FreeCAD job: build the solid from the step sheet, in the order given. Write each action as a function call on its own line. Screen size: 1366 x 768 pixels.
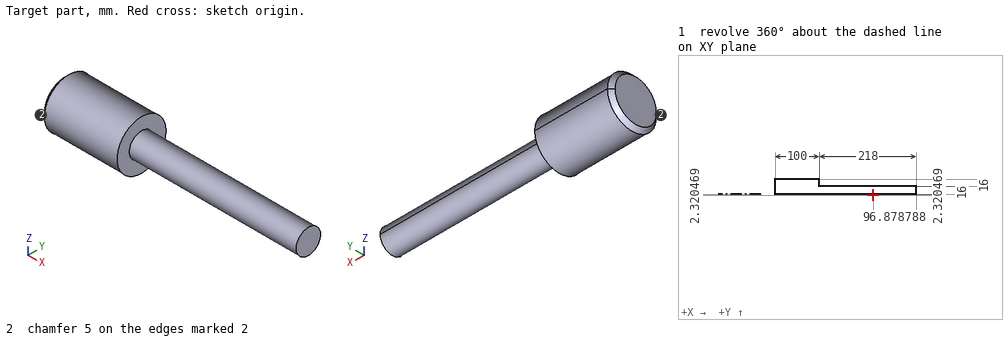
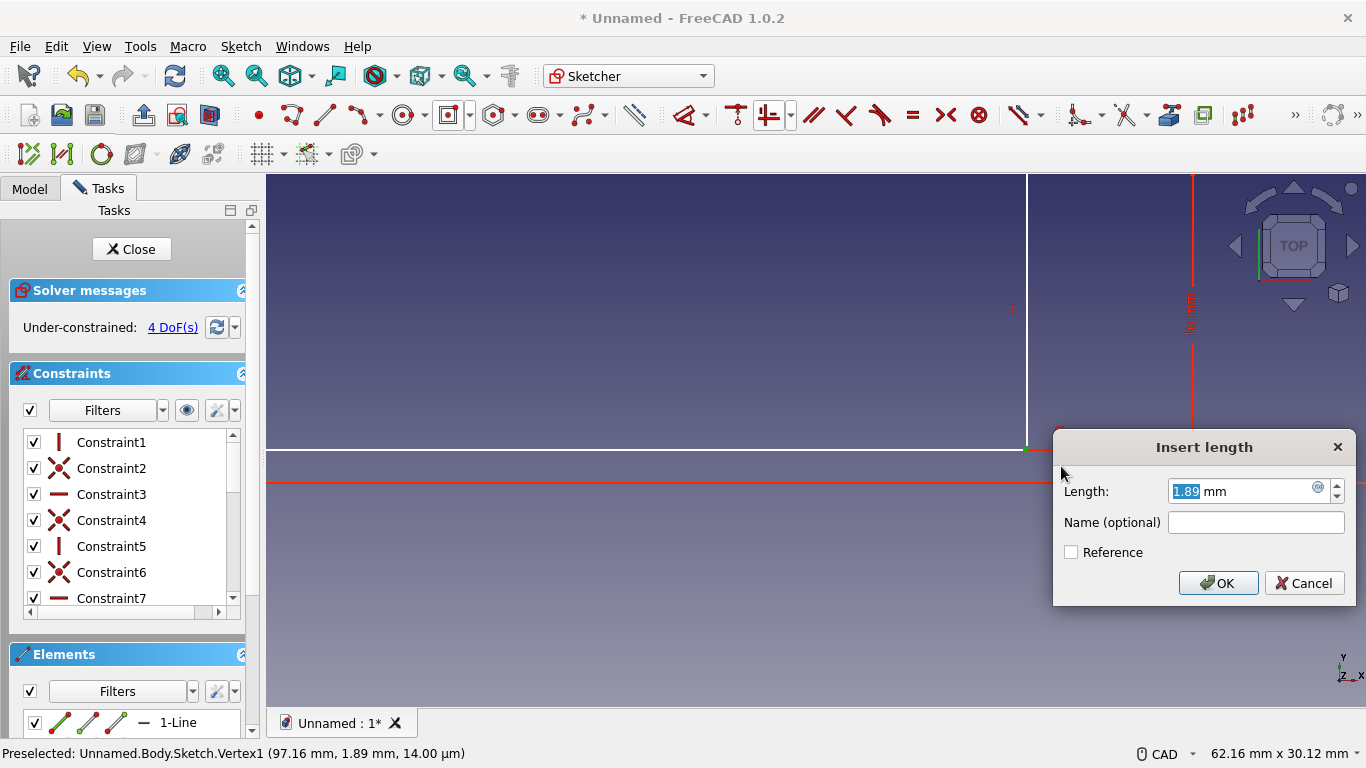
text(2.320469)
key(Return)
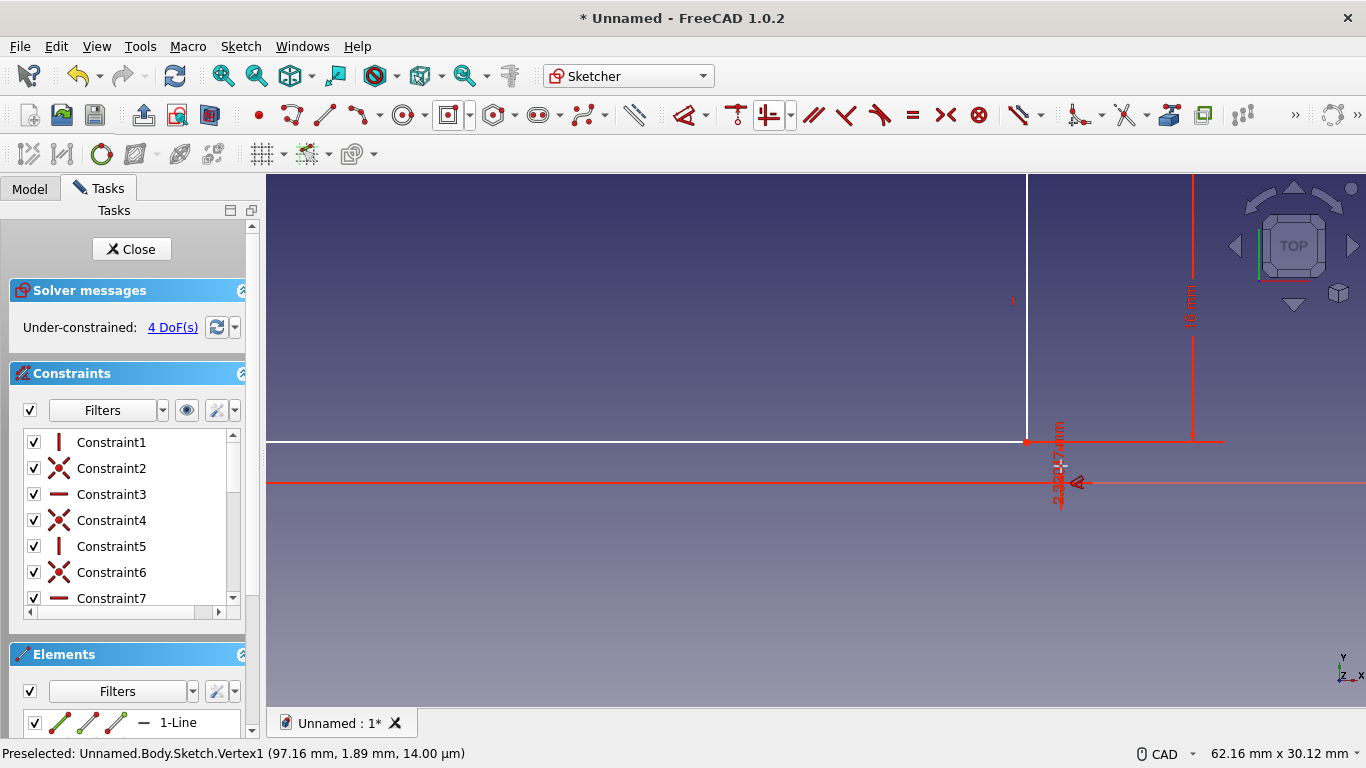
scroll(1042, 461, down, 13)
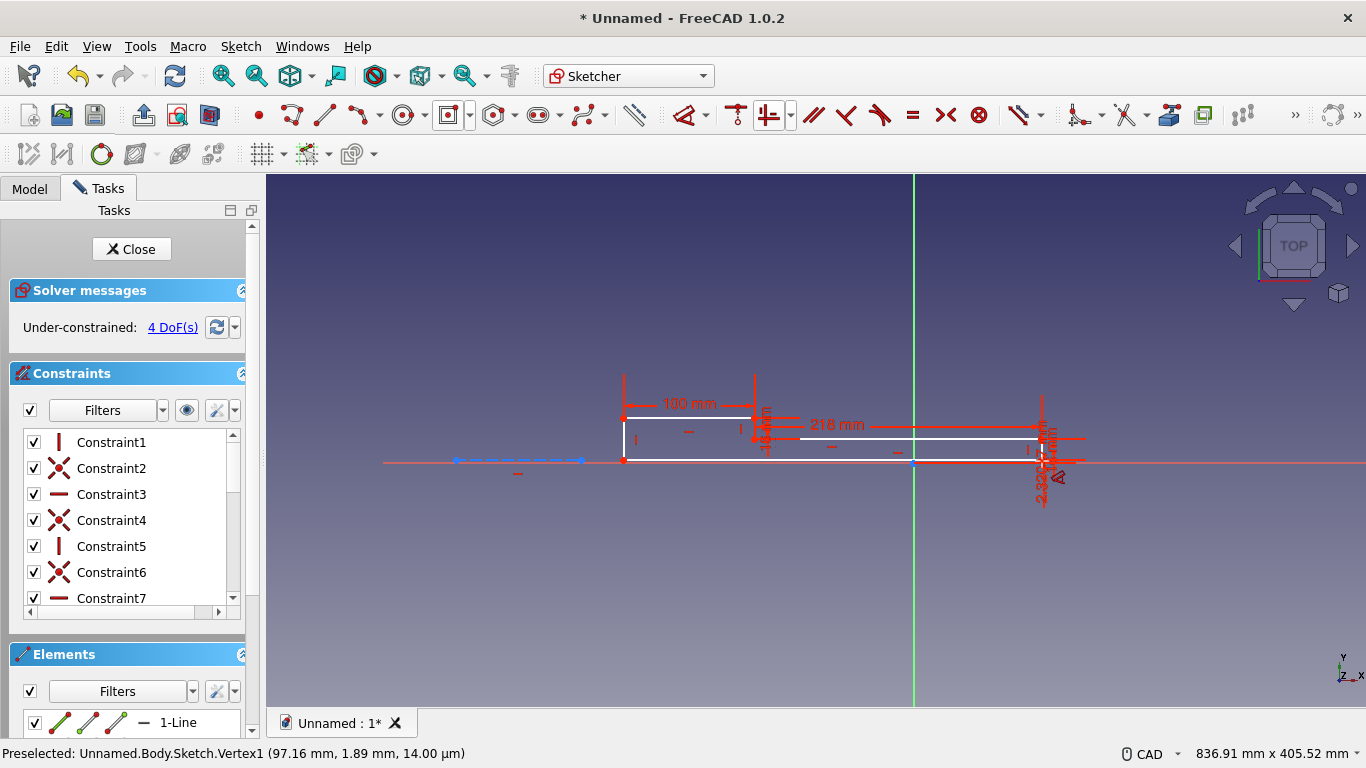
scroll(581, 460, up, 13)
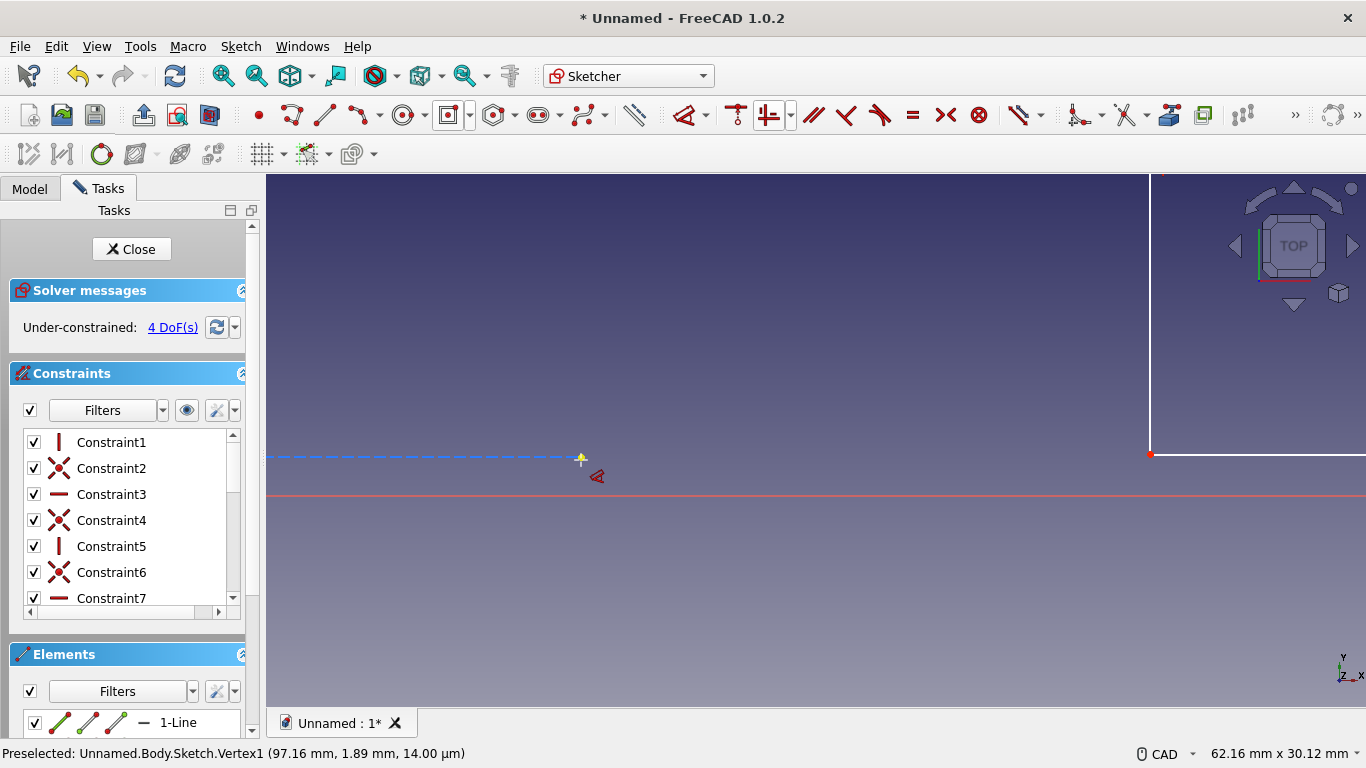
click(582, 457)
click(548, 476)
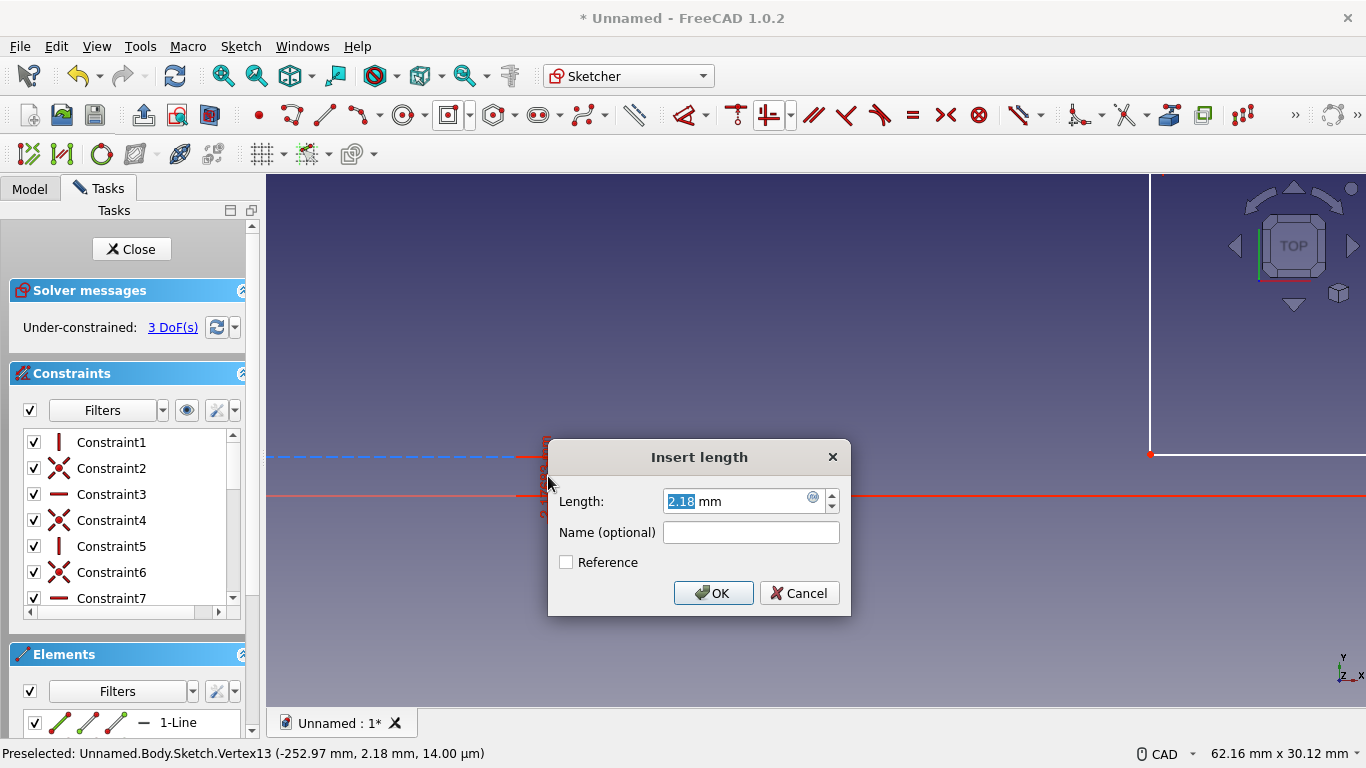
text(2.320469)
key(Return)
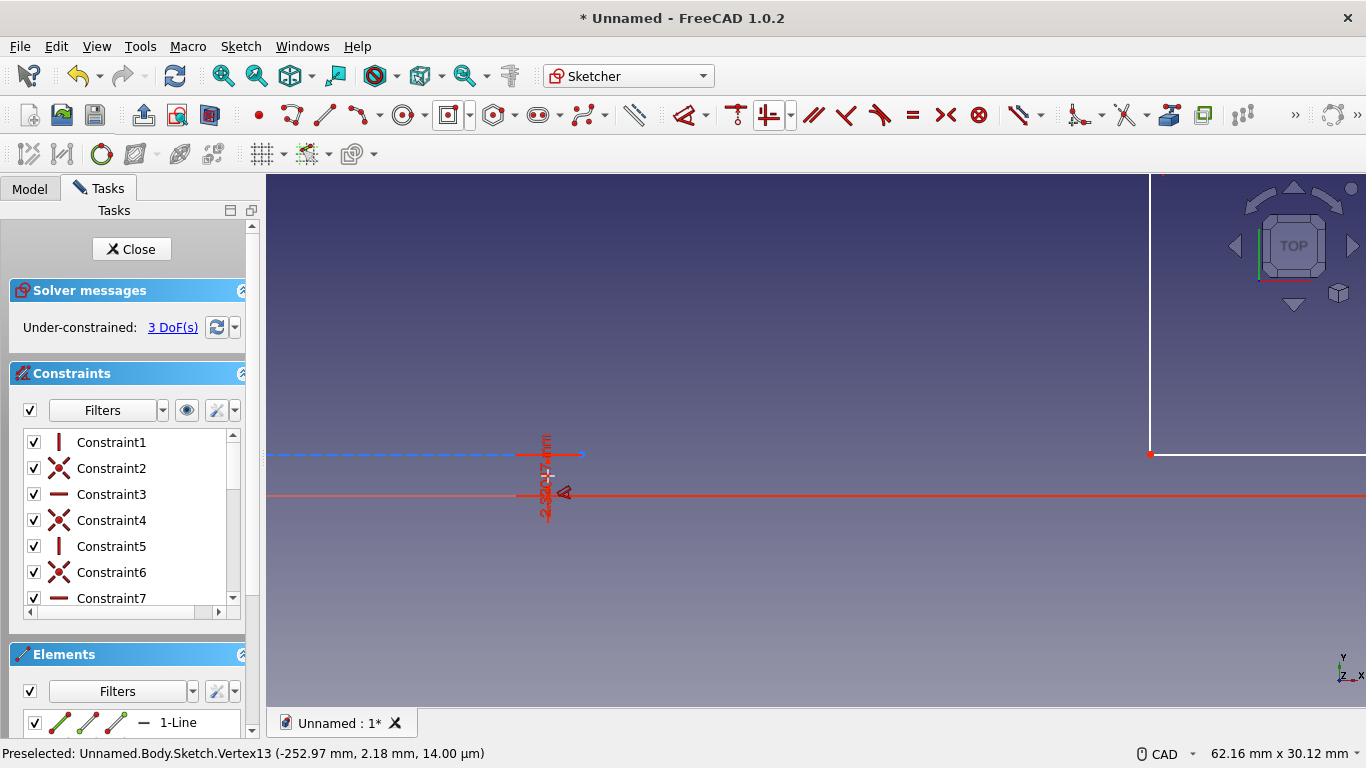
scroll(580, 460, down, 13)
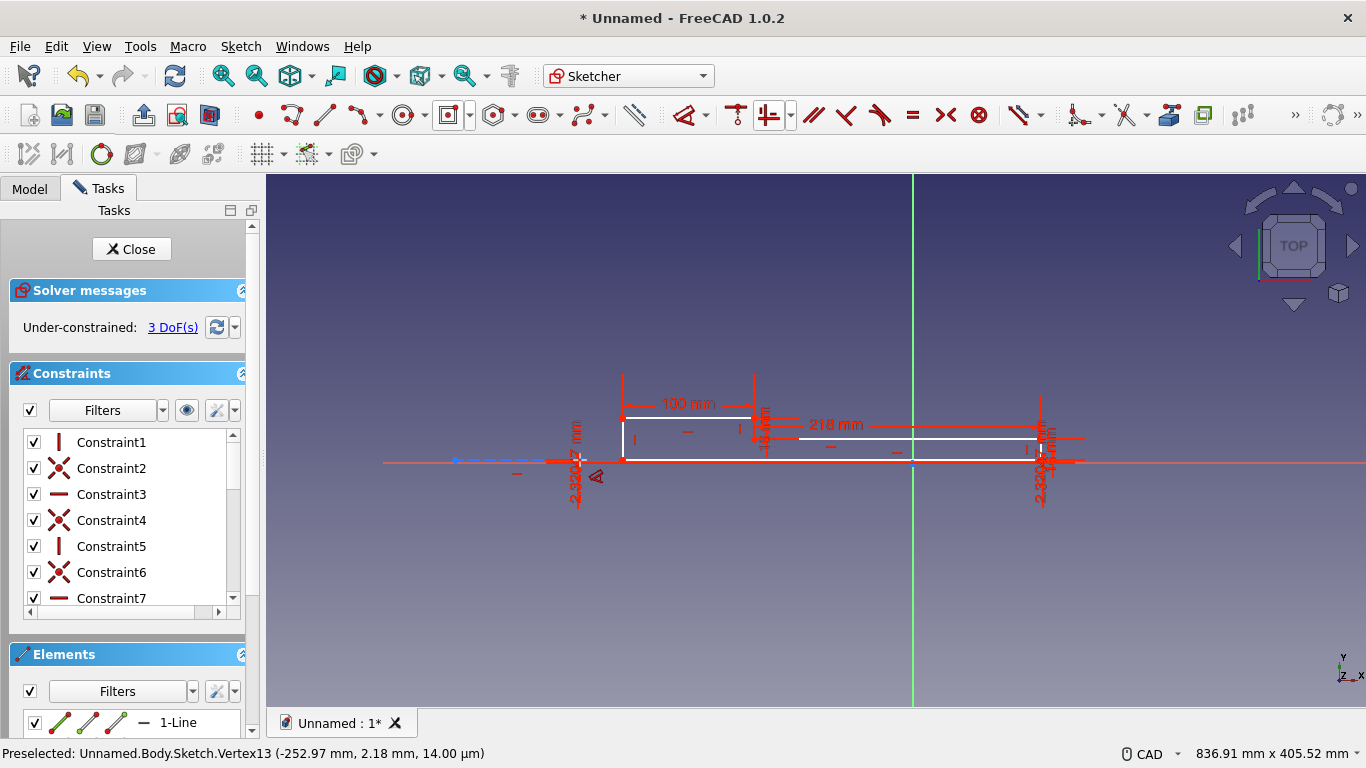
click(1041, 460)
click(977, 497)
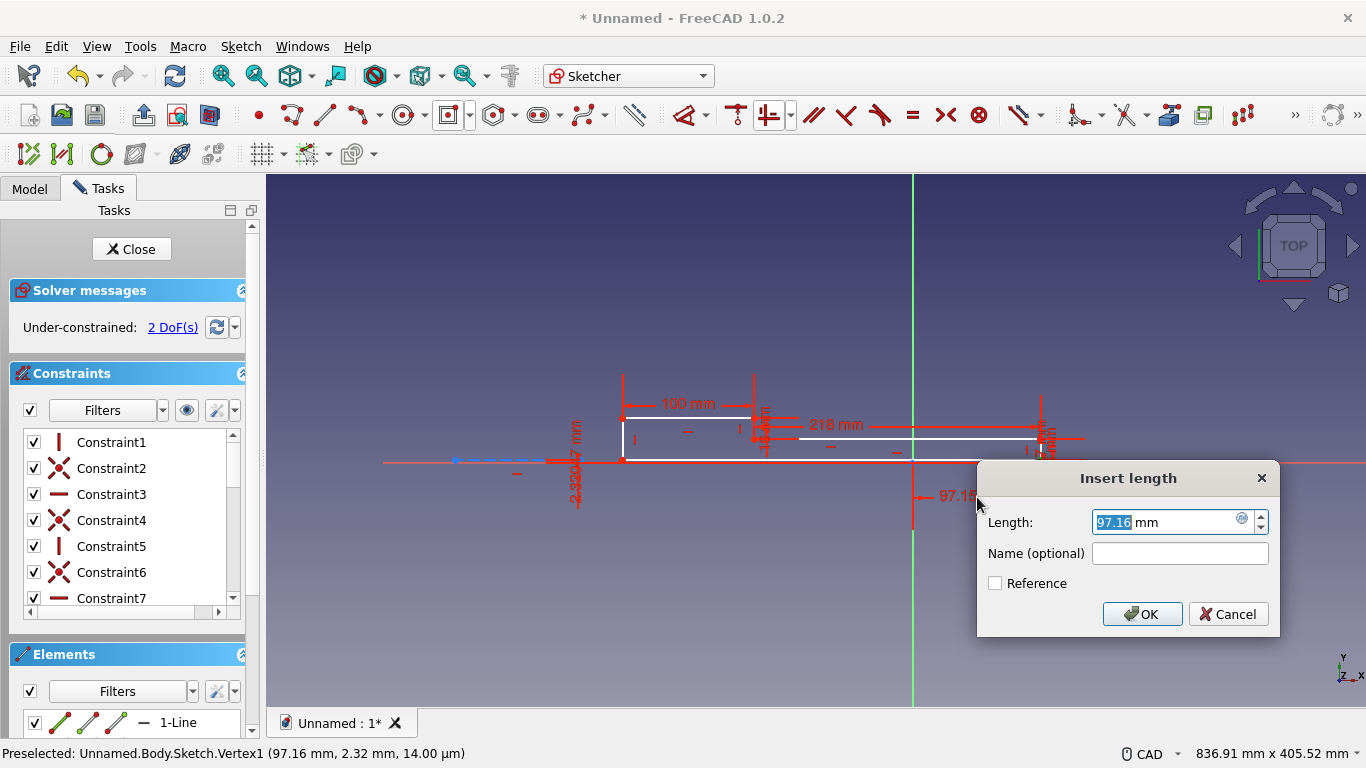
text(96.878788)
key(Return)
key(Escape)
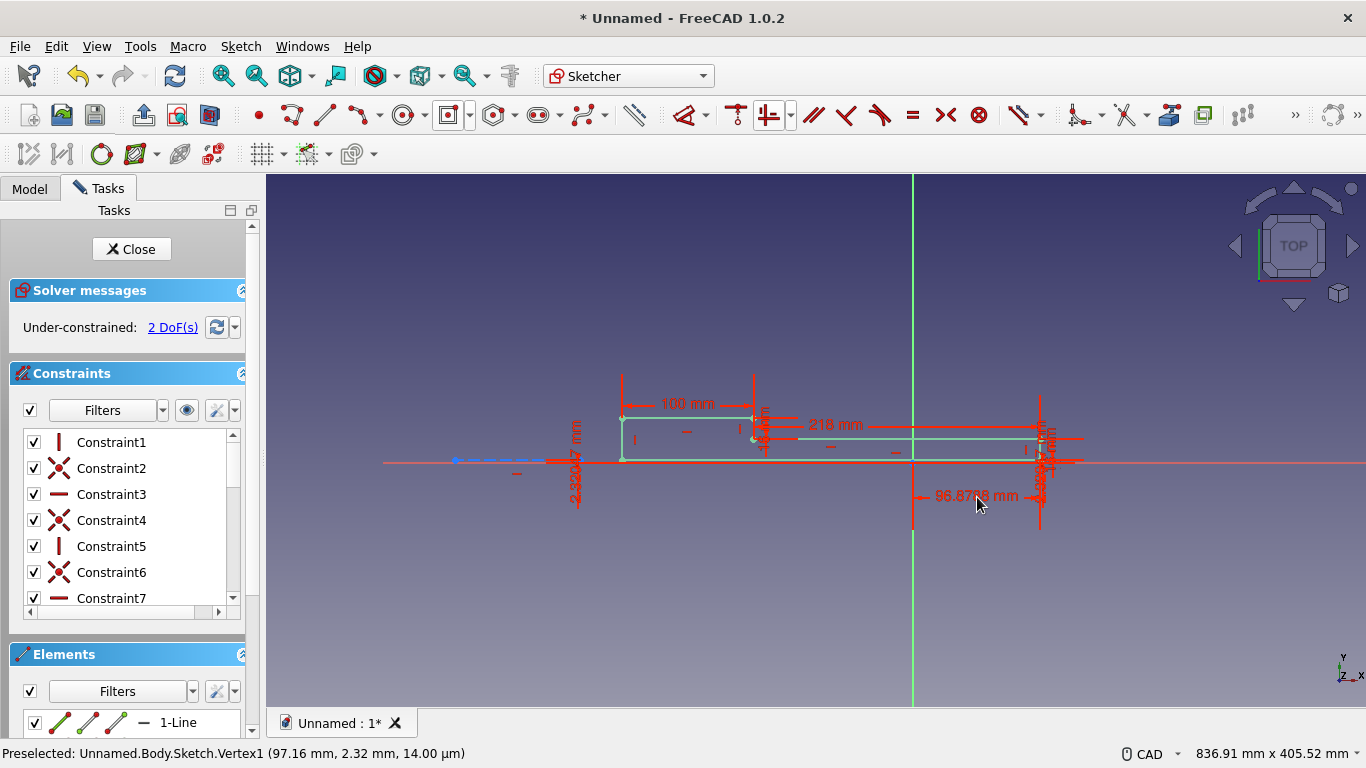
click(132, 249)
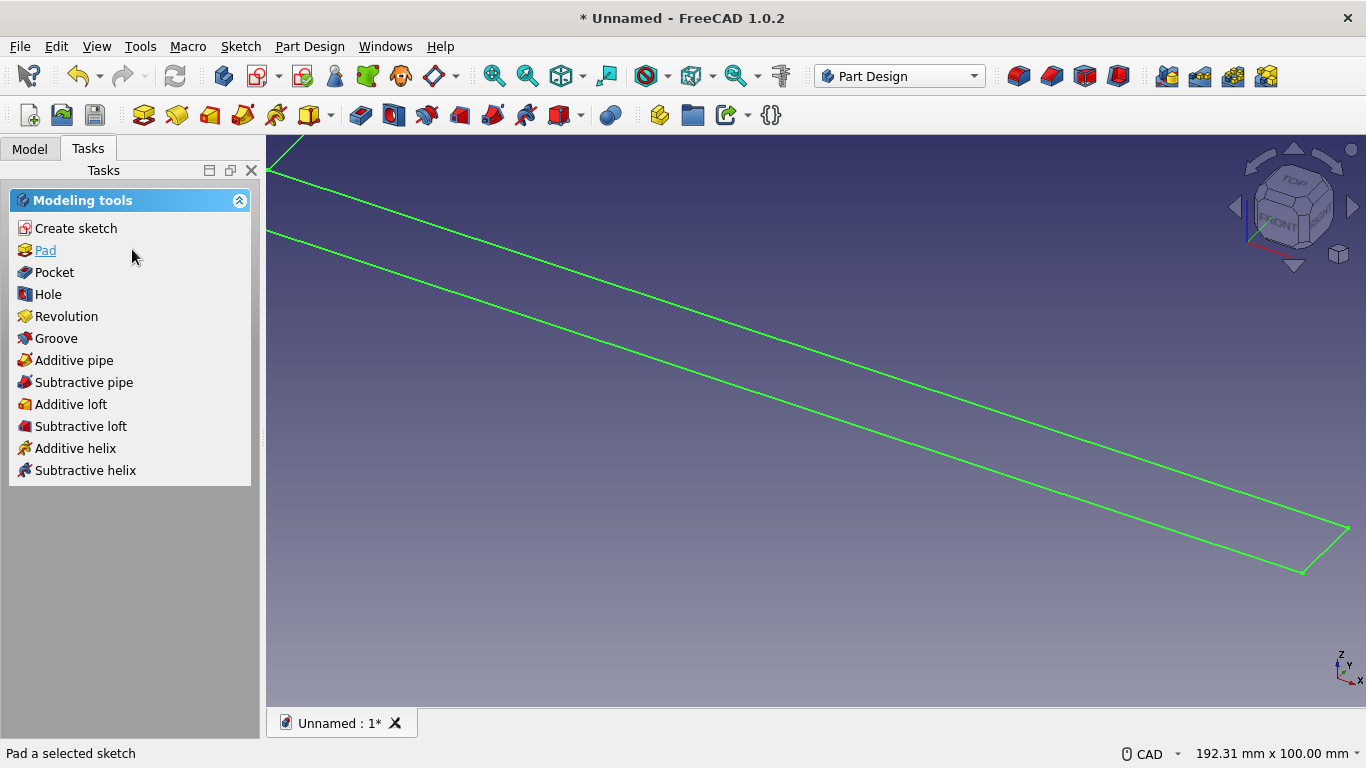
click(177, 116)